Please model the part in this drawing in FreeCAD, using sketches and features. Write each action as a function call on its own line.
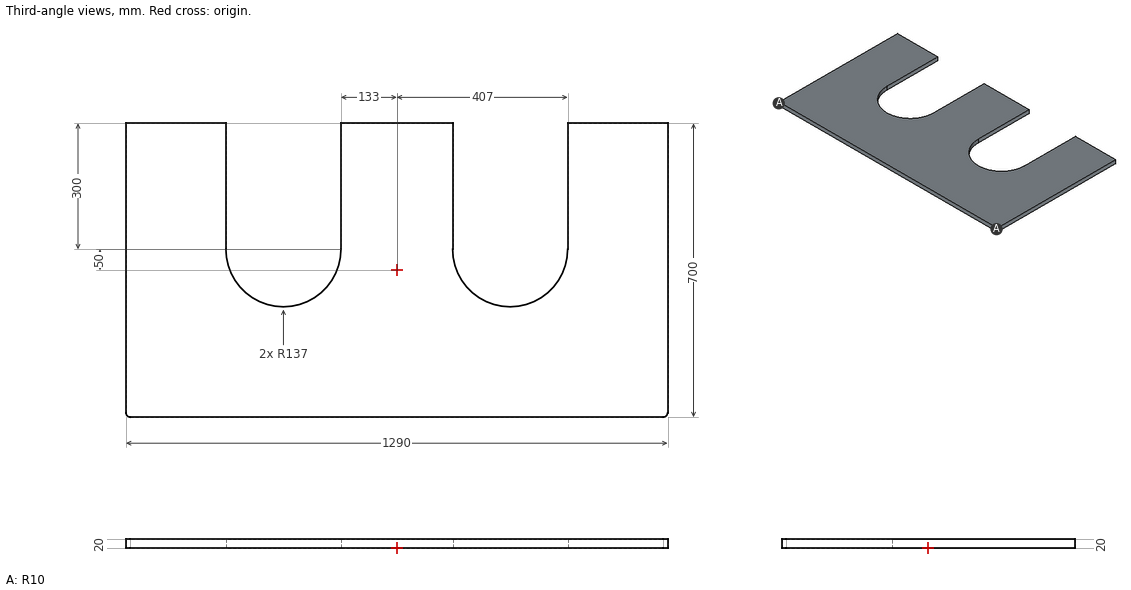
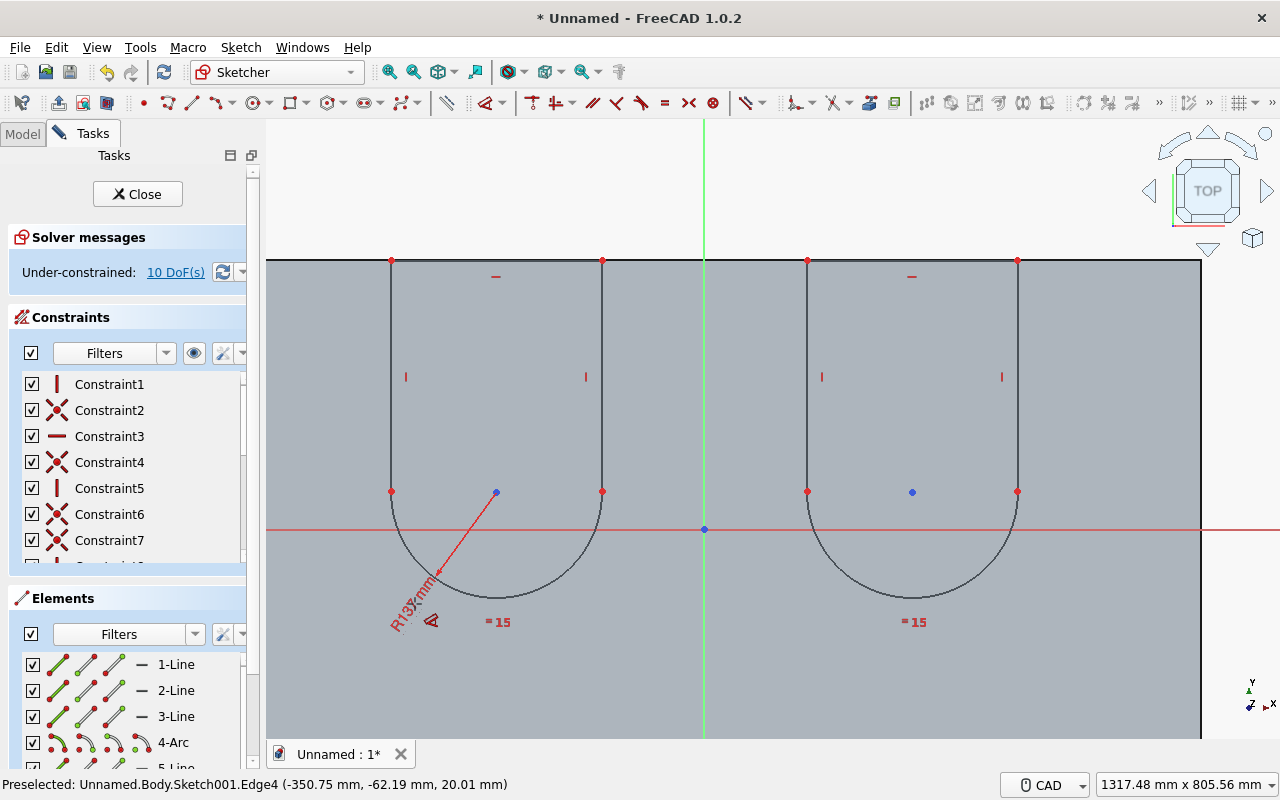
click(602, 423)
click(568, 376)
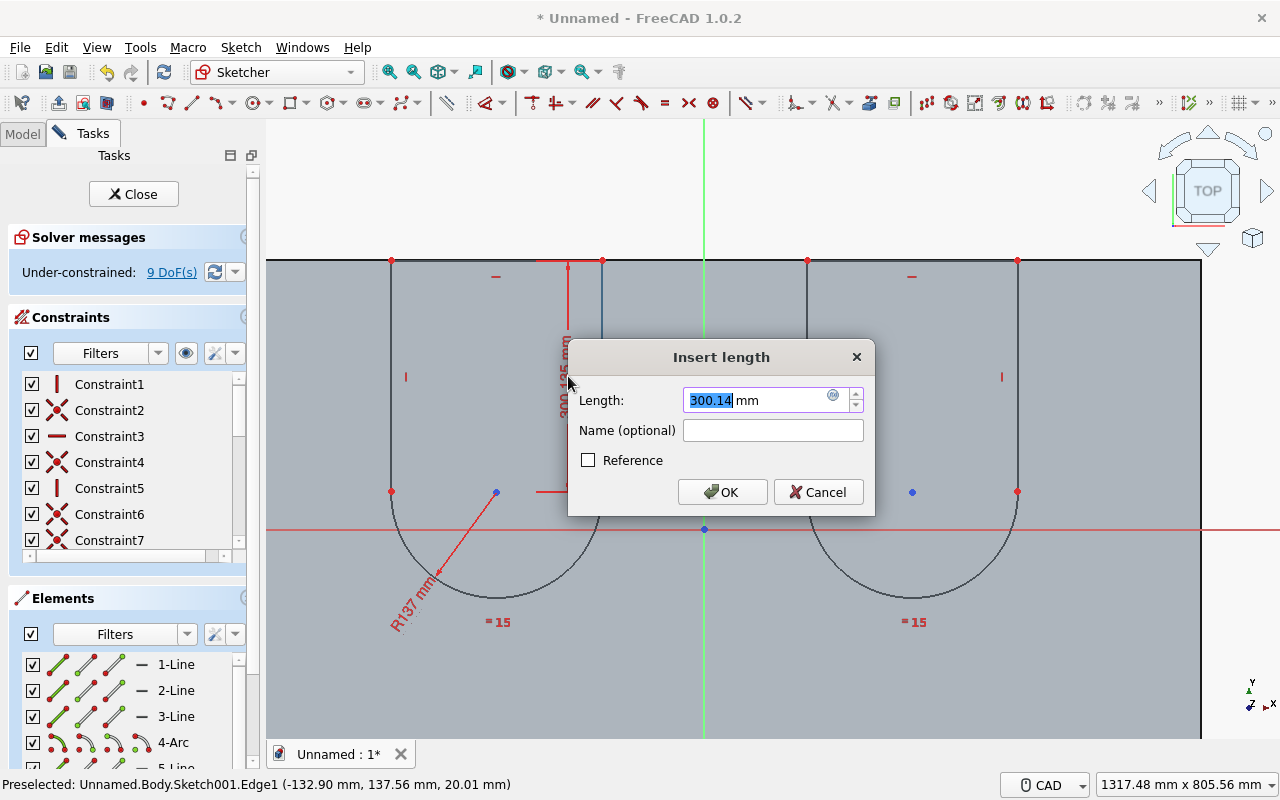
text(300)
key(Return)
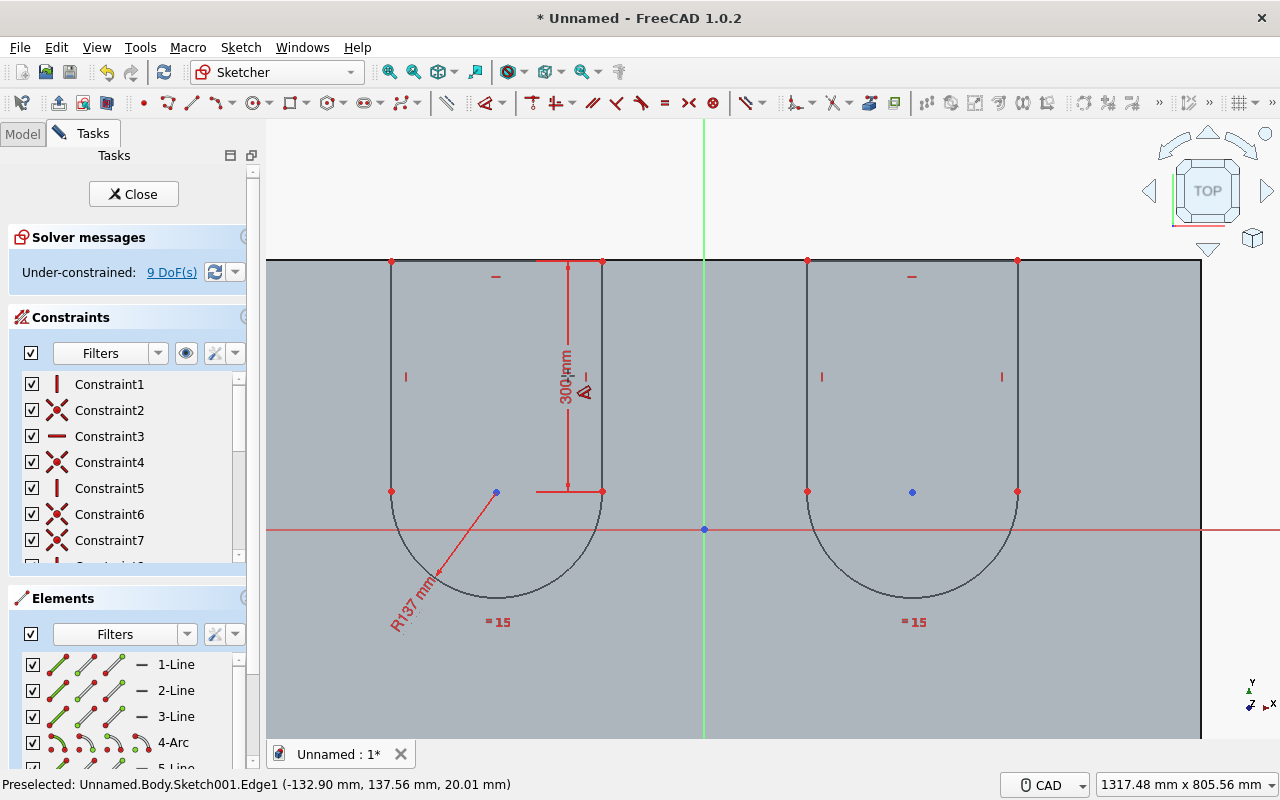
click(391, 330)
click(357, 377)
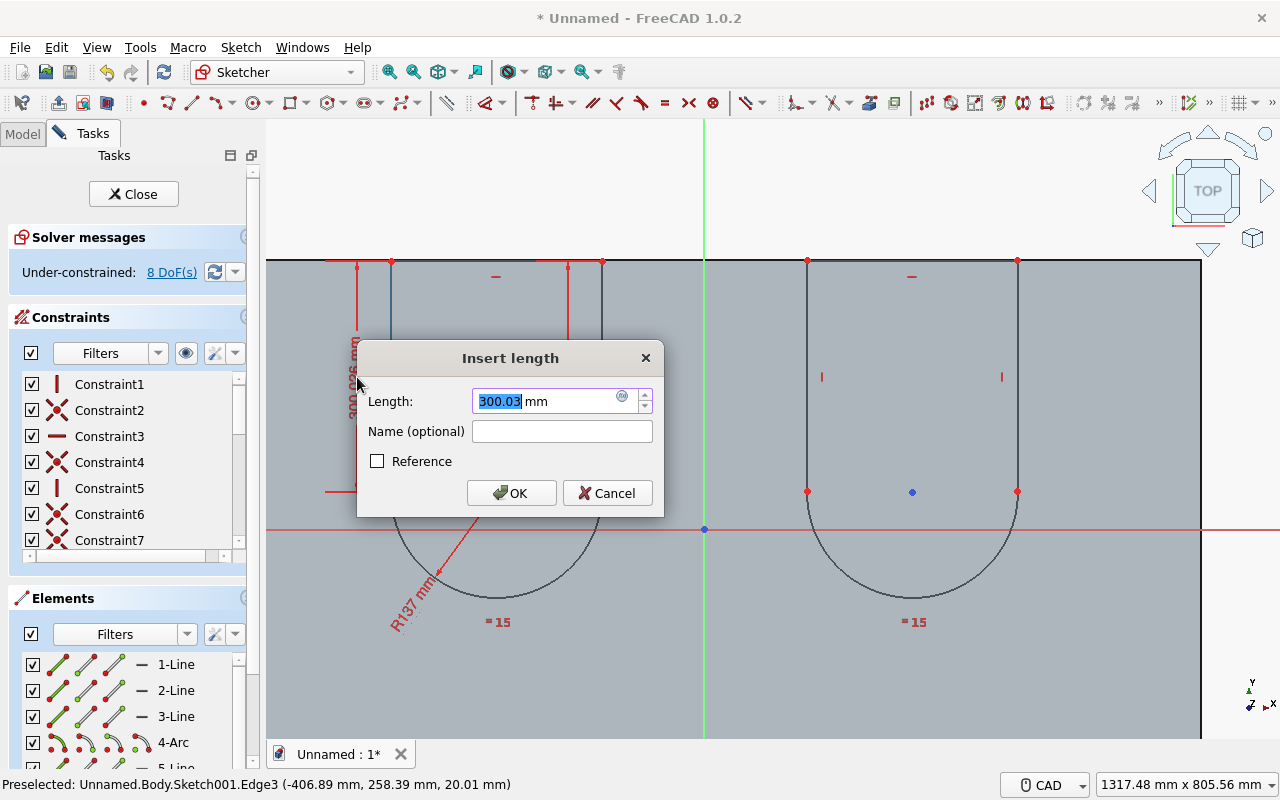
text(300)
key(Return)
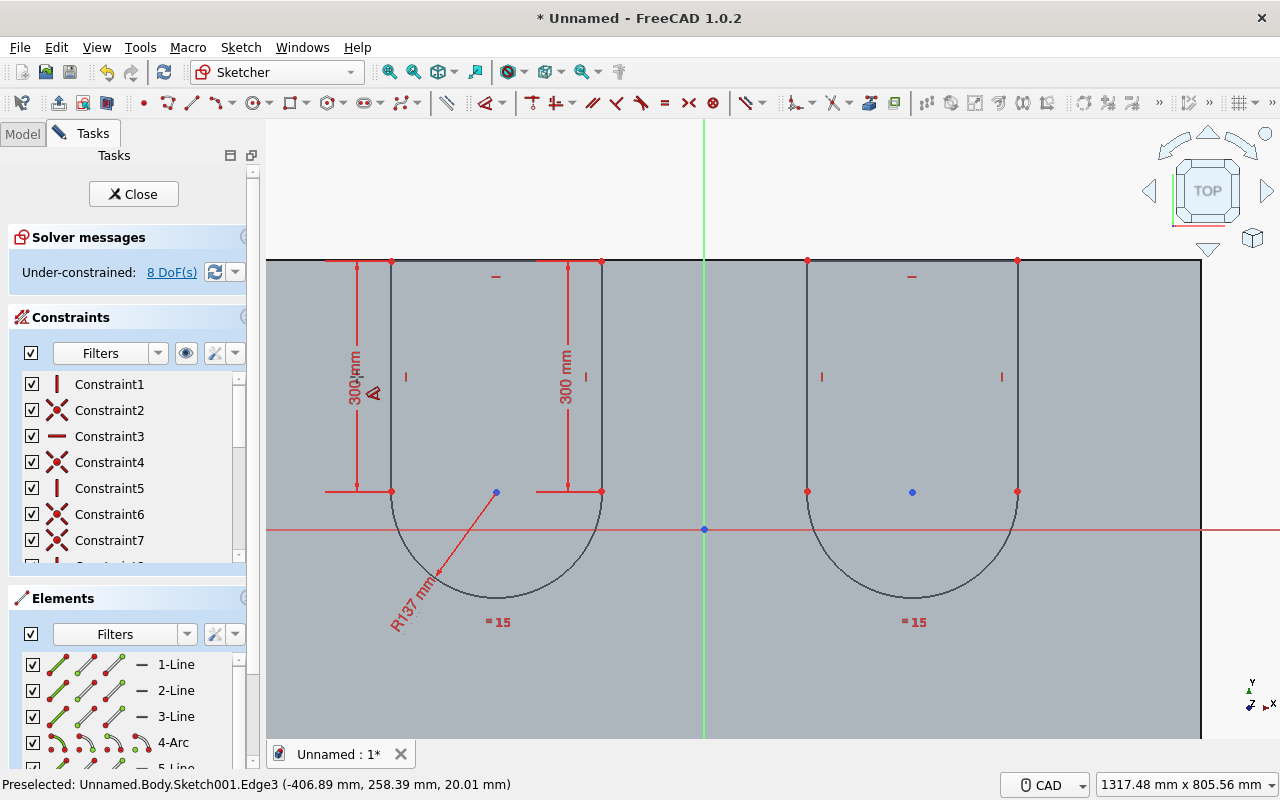
click(1018, 423)
click(1052, 377)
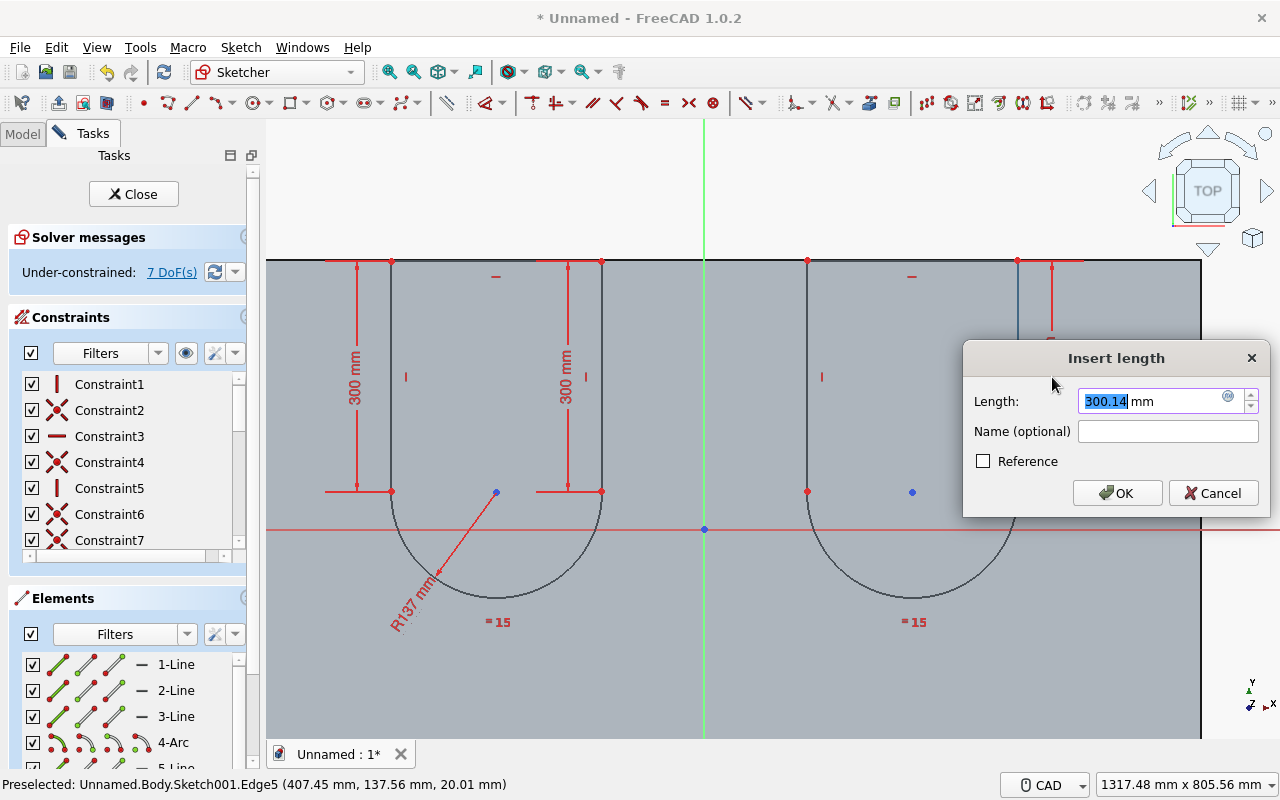
text(300)
key(Return)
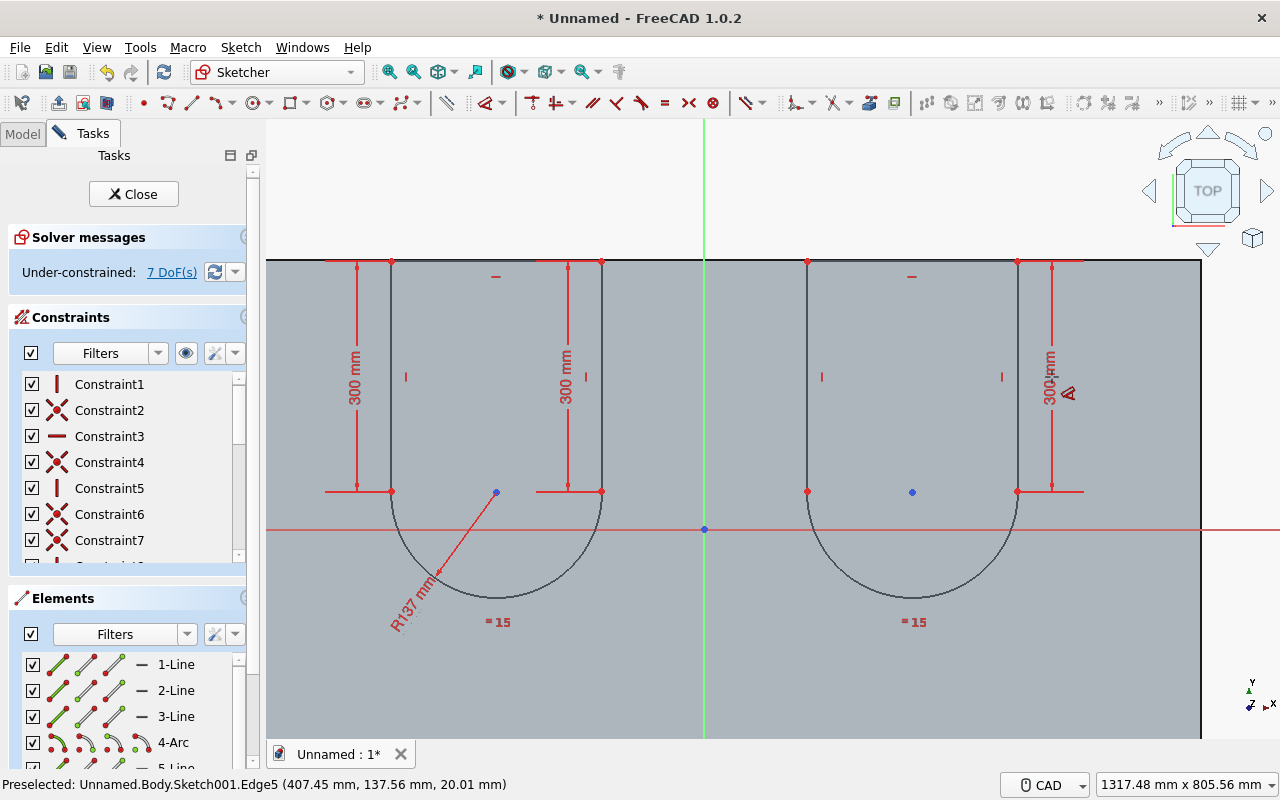
click(807, 330)
click(841, 377)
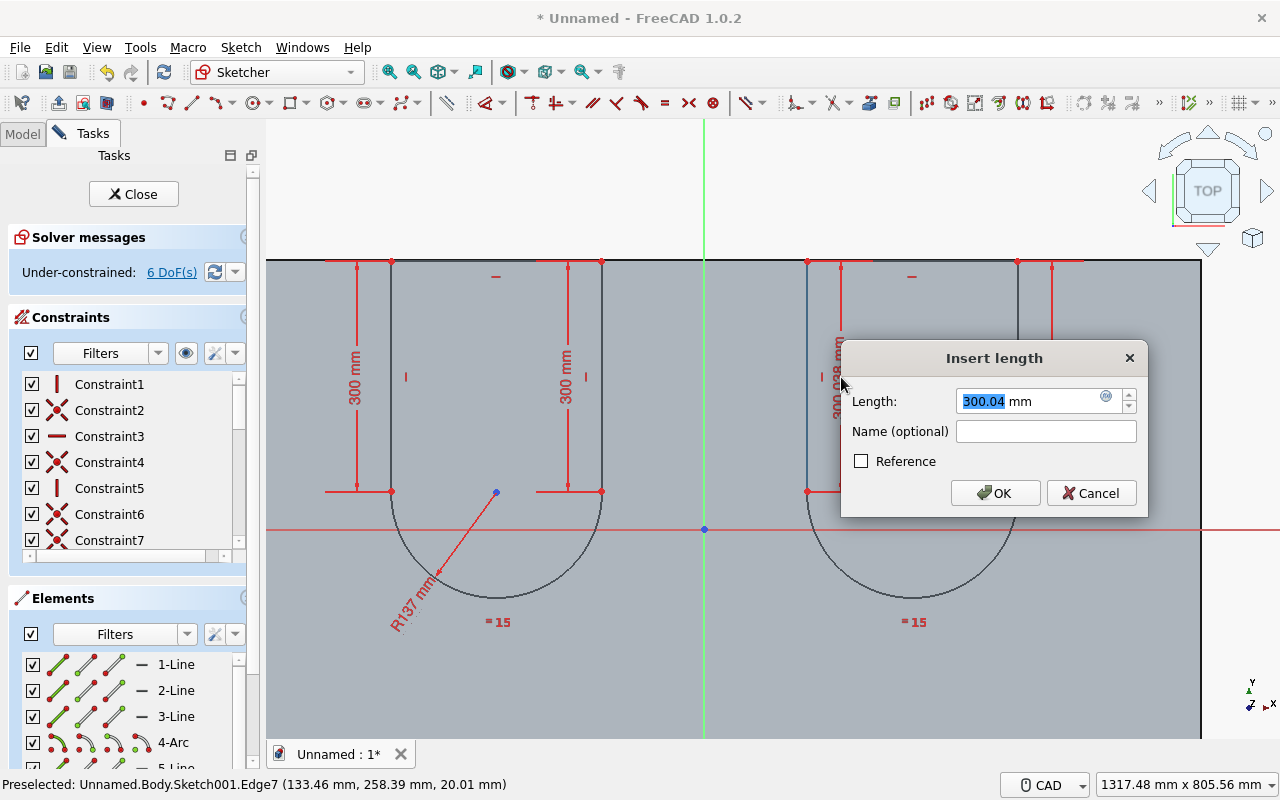
text(300)
key(Return)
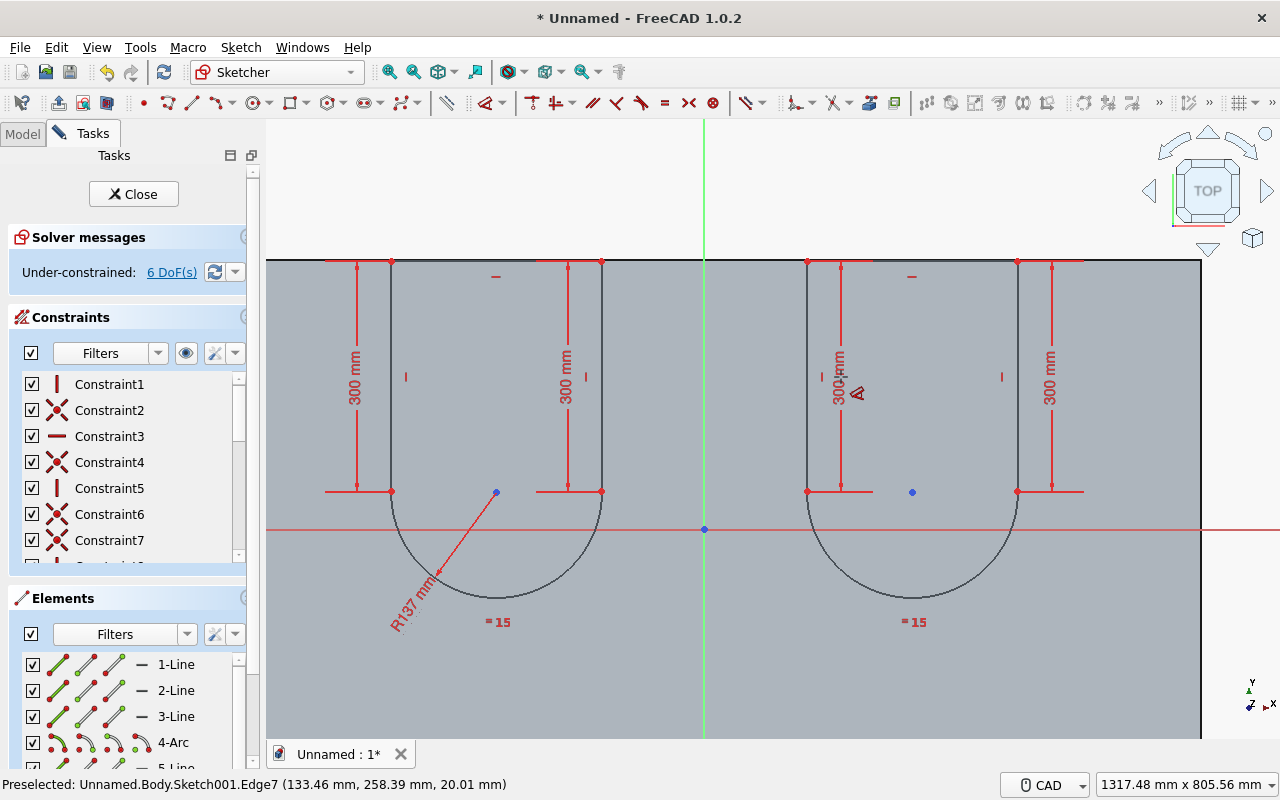
click(602, 492)
click(568, 511)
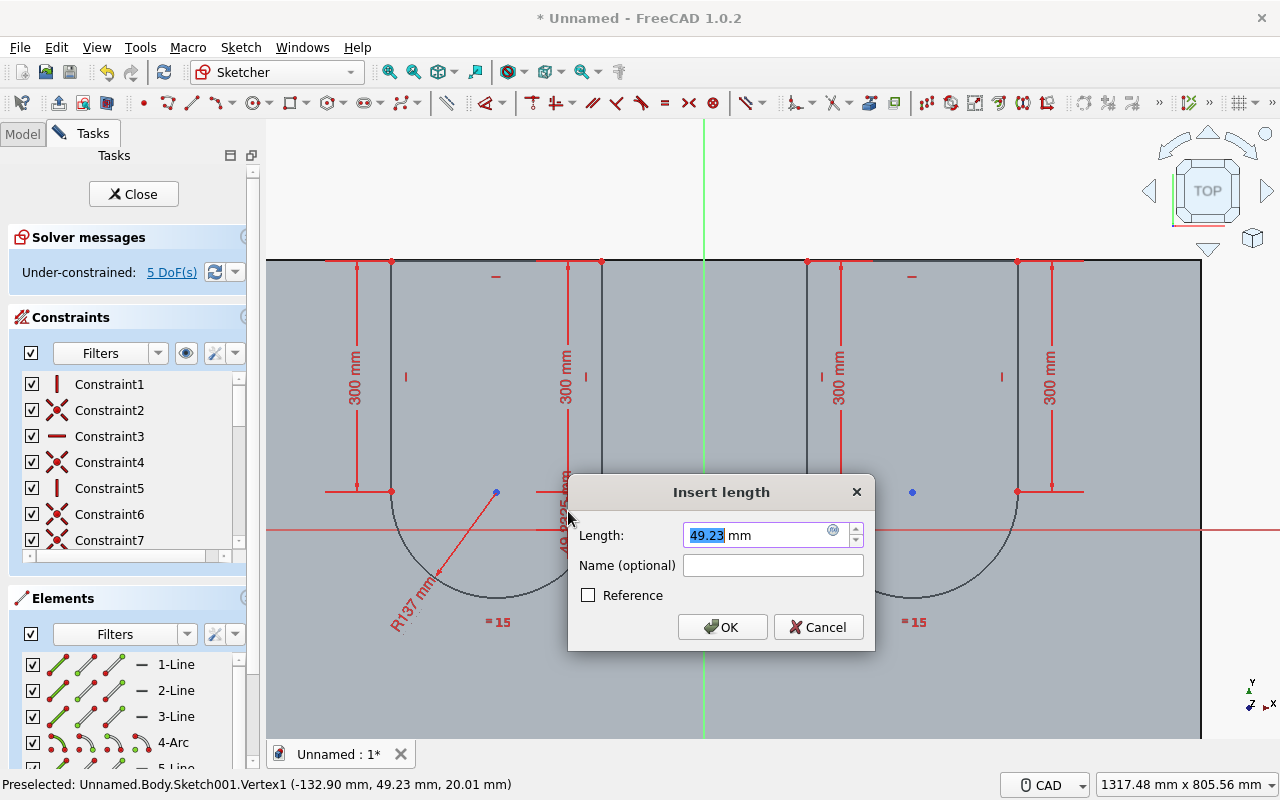
text(50)
key(Return)